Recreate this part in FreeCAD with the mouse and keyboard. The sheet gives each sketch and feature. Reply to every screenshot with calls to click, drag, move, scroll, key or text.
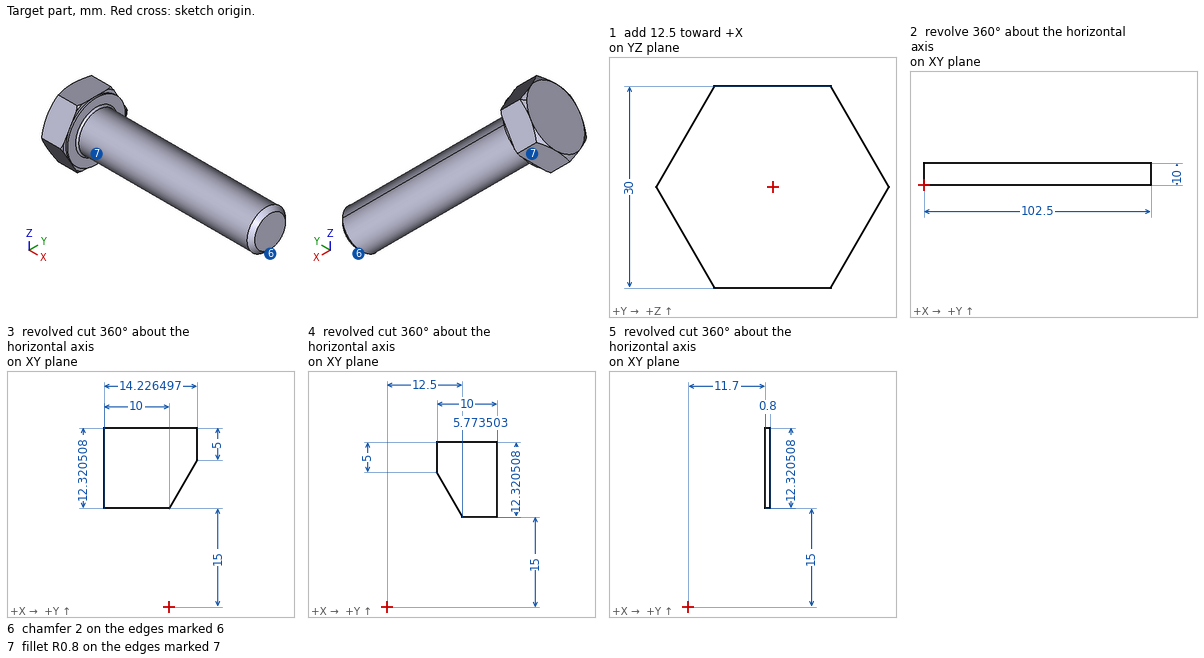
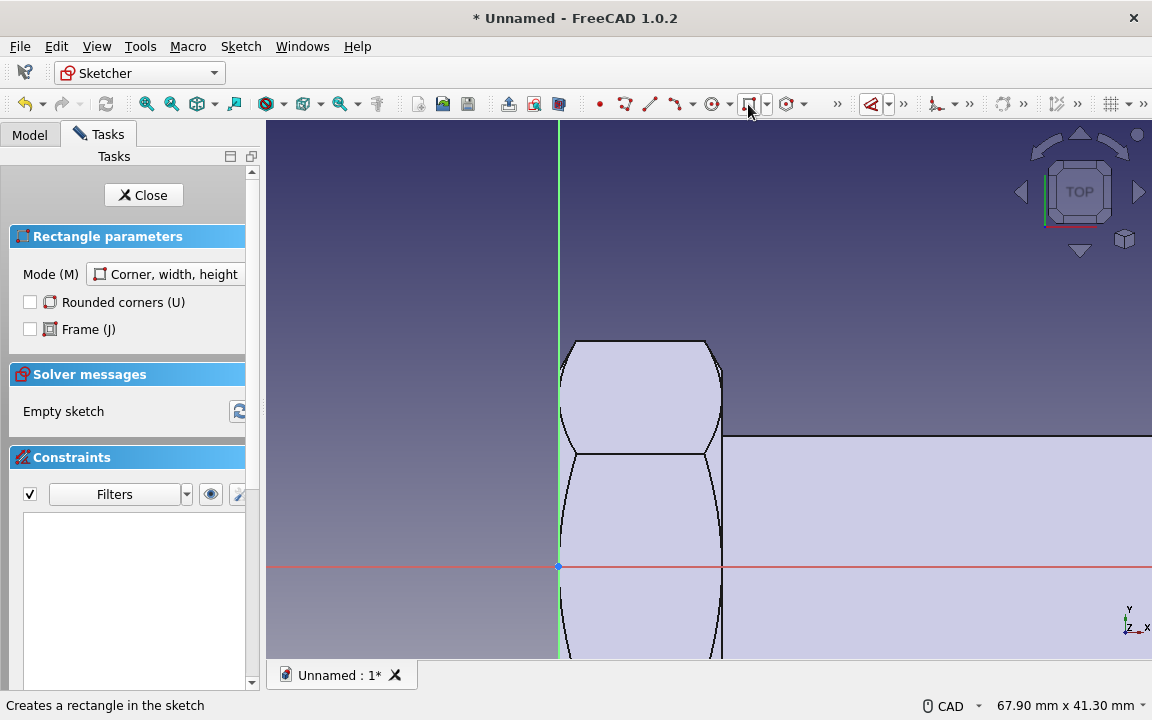
scroll(712, 210, up, 3)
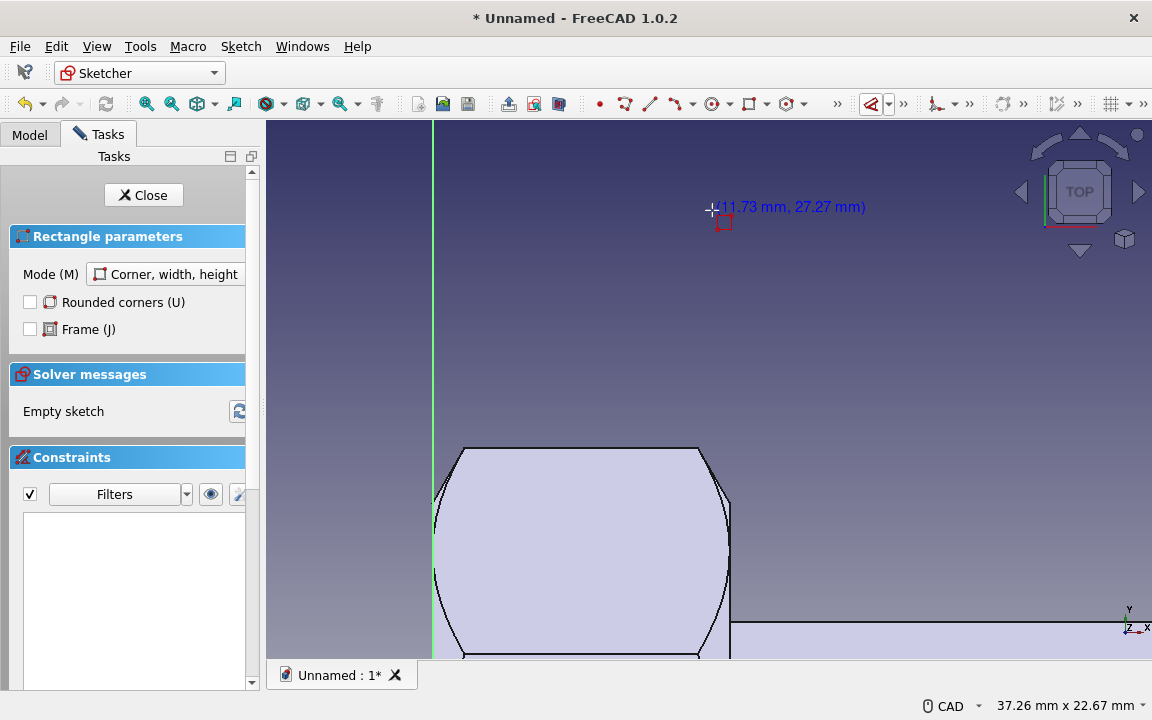
click(711, 210)
move(730, 503)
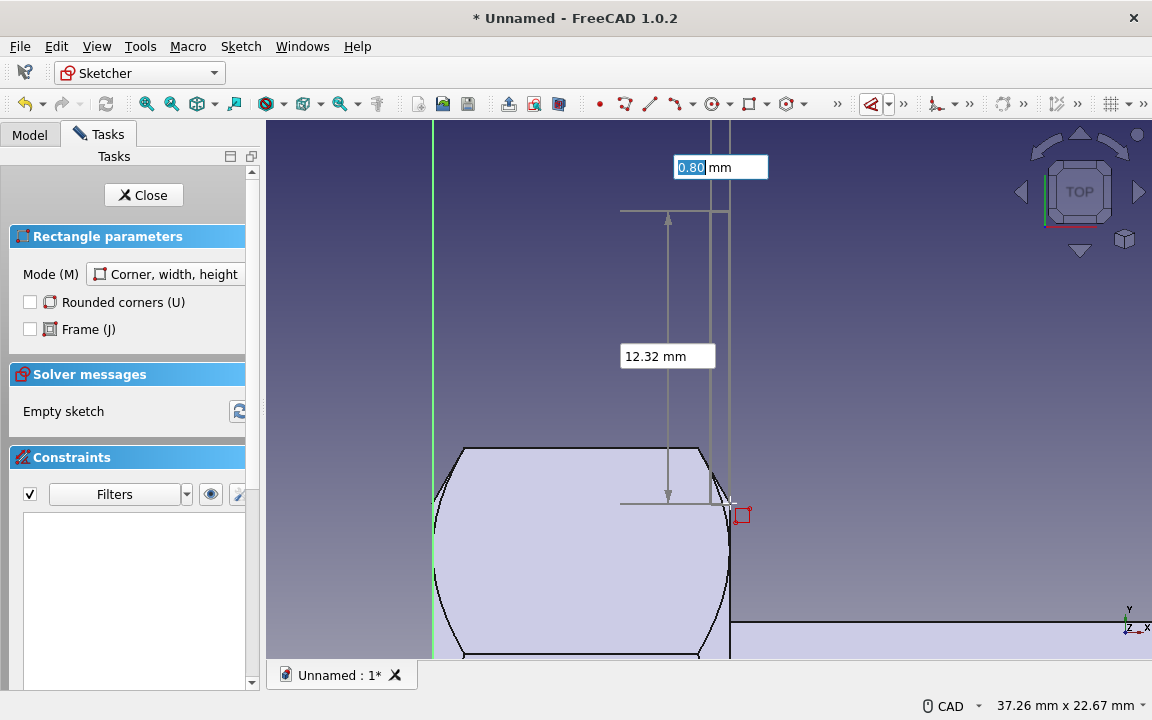
text(0.8)
key(Tab)
text(12.320508)
key(Return)
key(Escape)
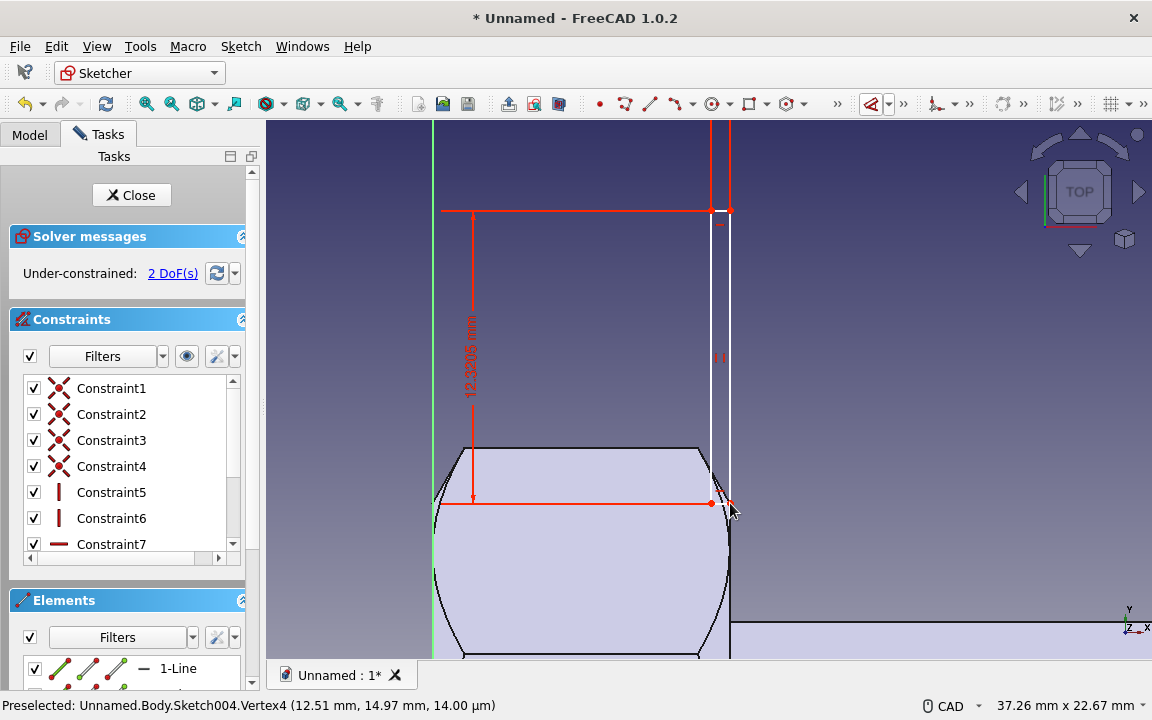
click(711, 504)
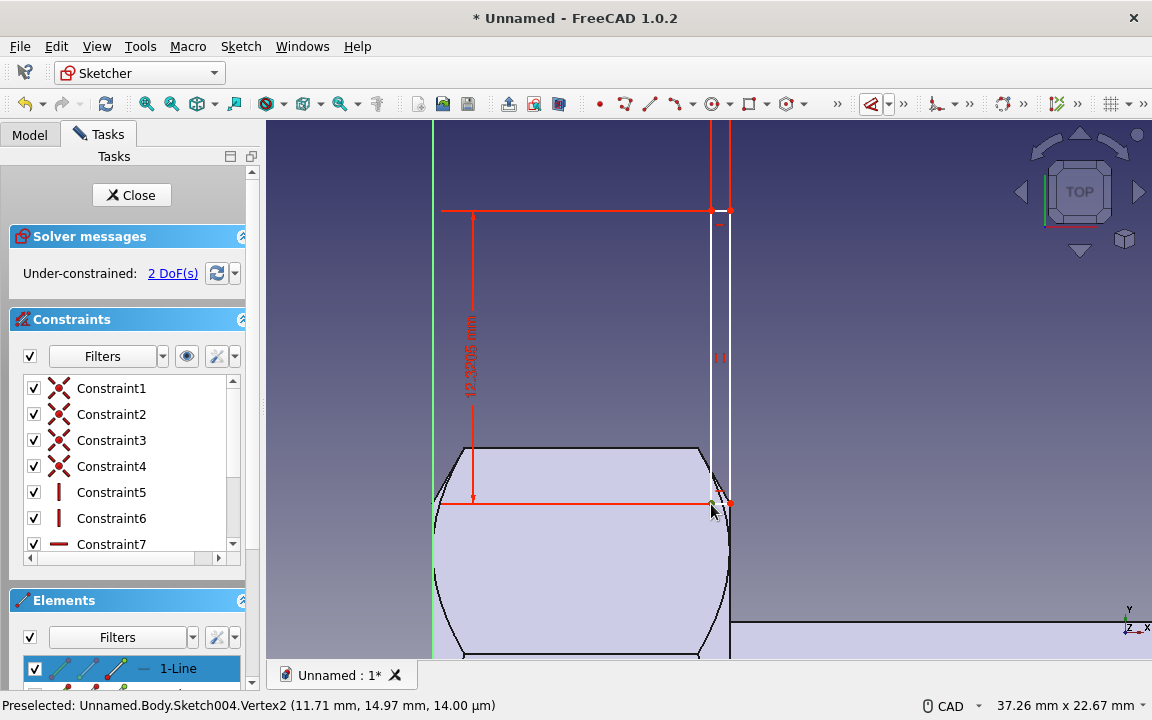
click(888, 104)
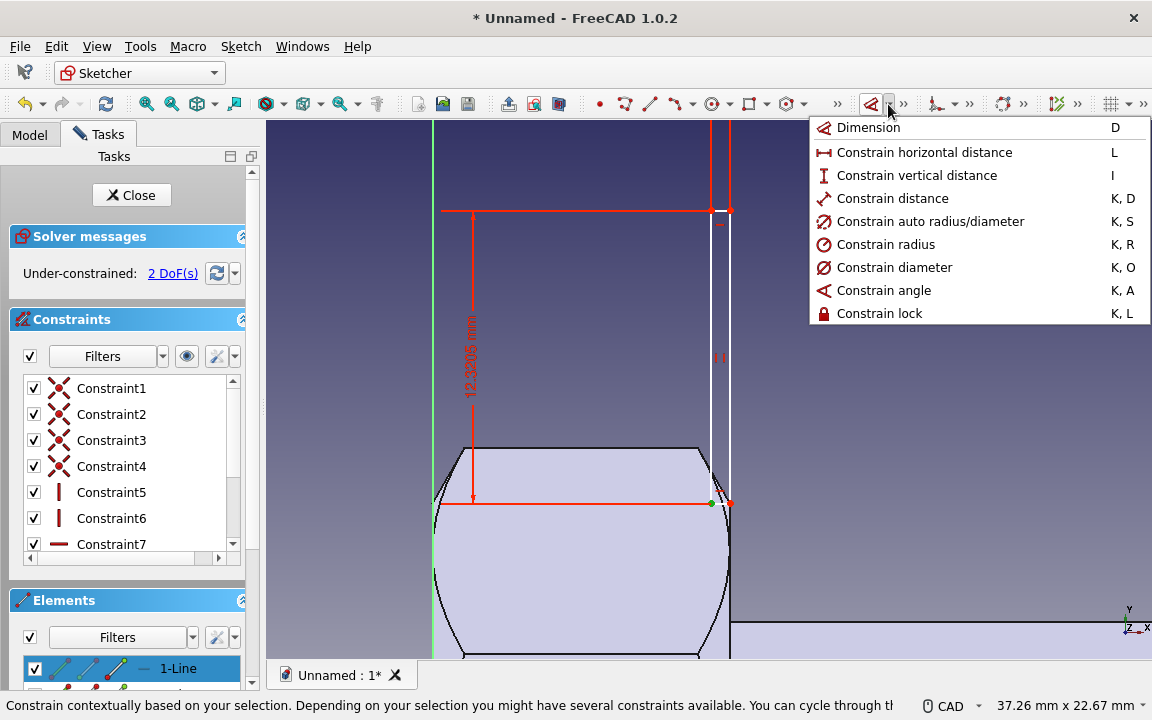
click(980, 176)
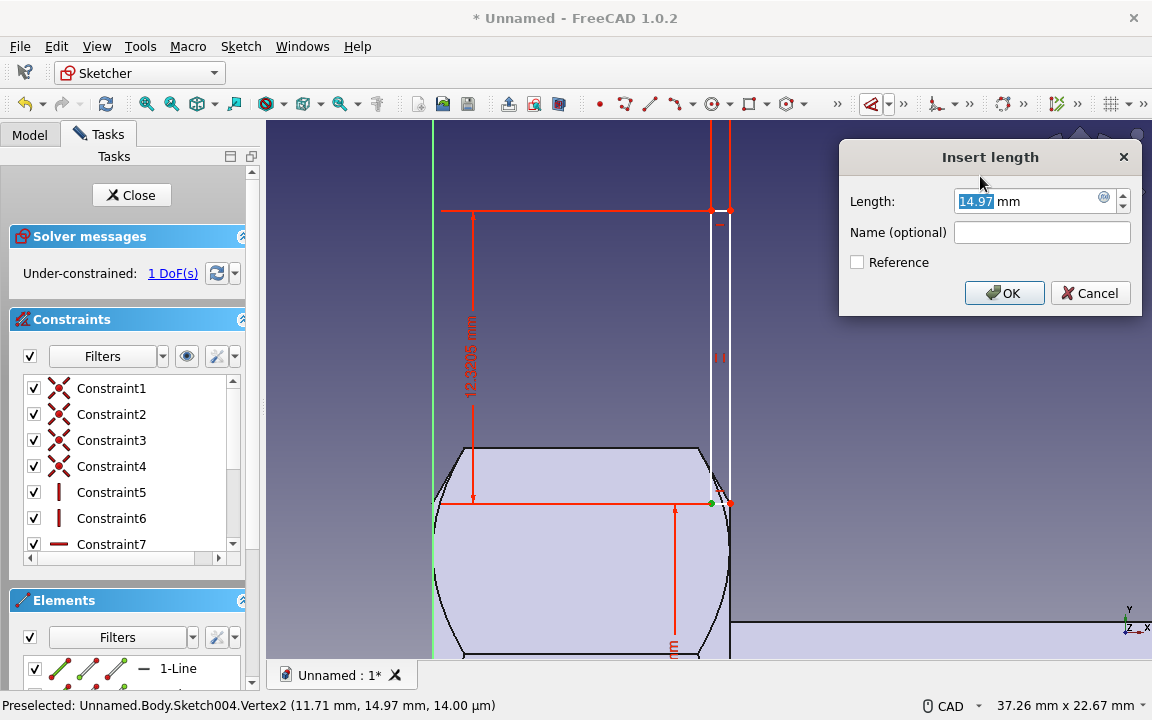
text(15)
key(Return)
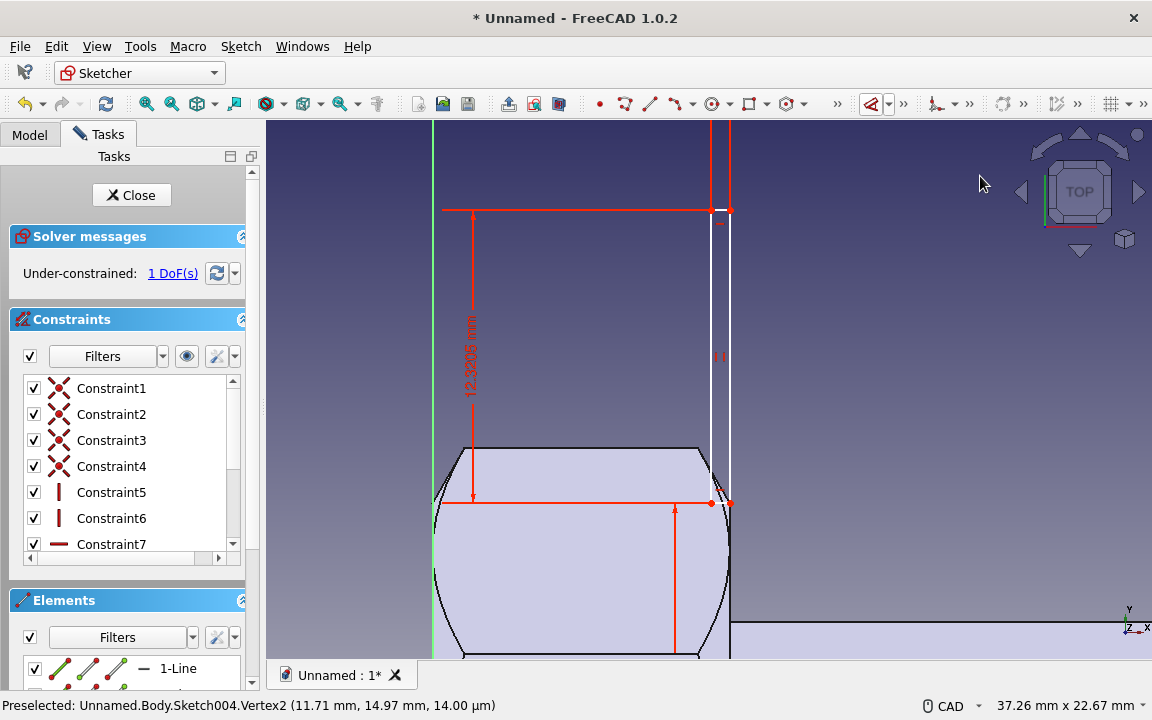
click(711, 210)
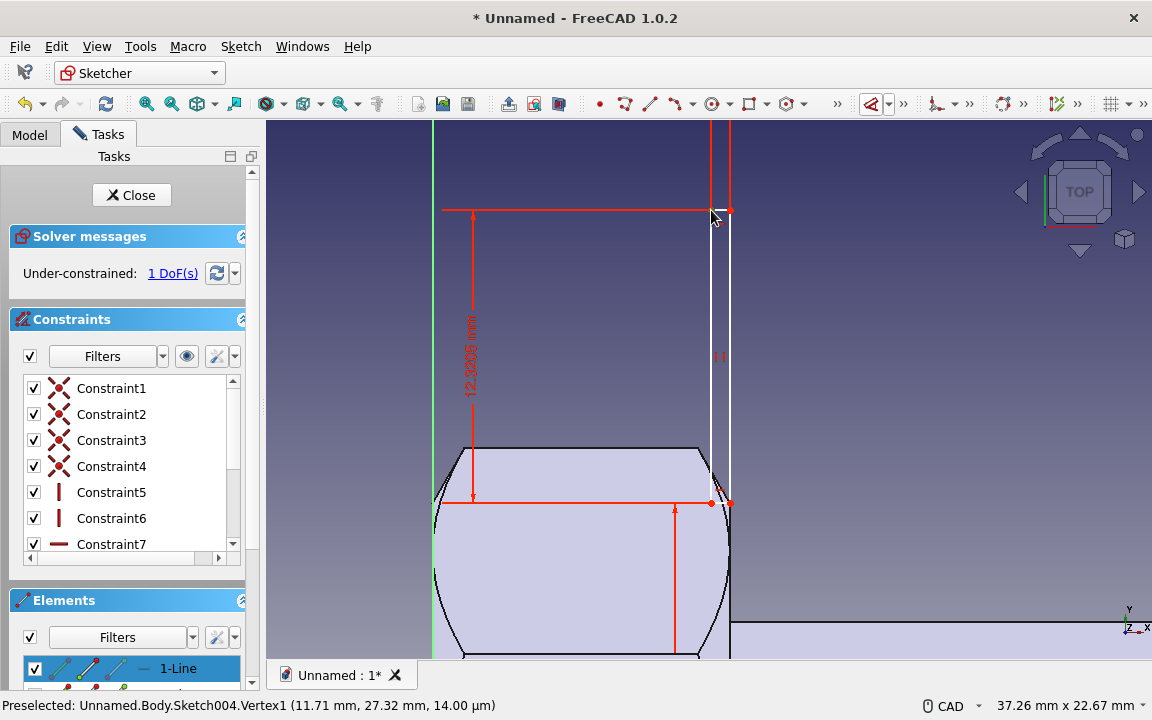
click(888, 104)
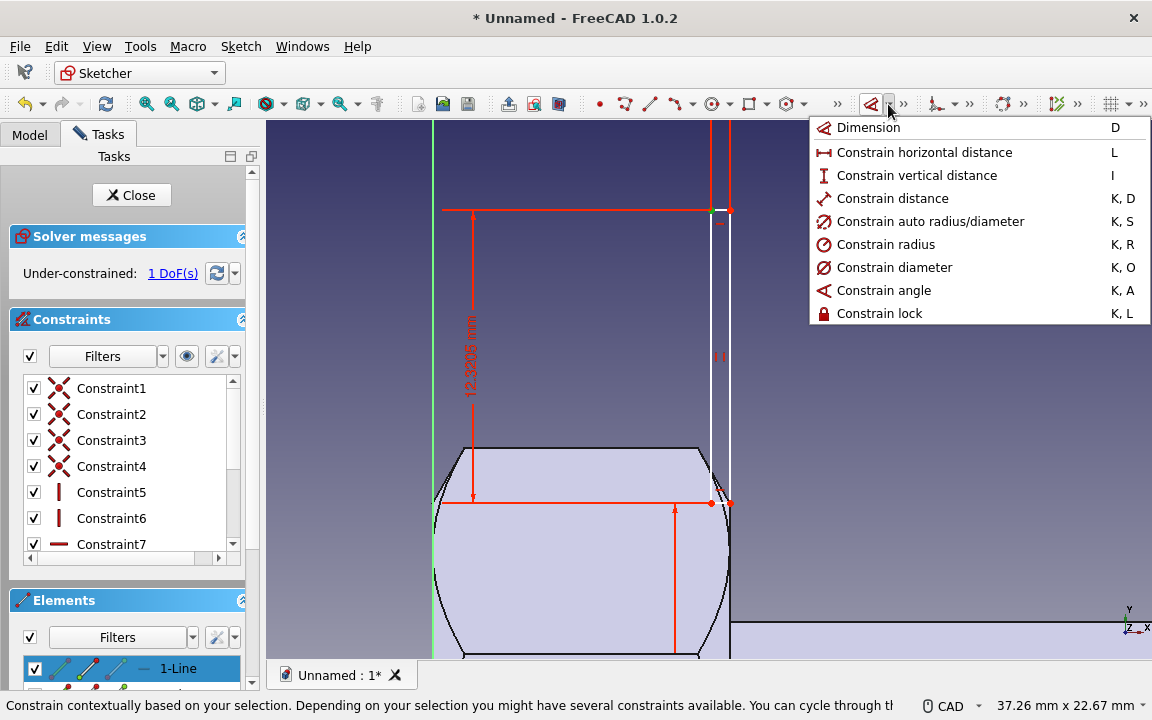
click(980, 152)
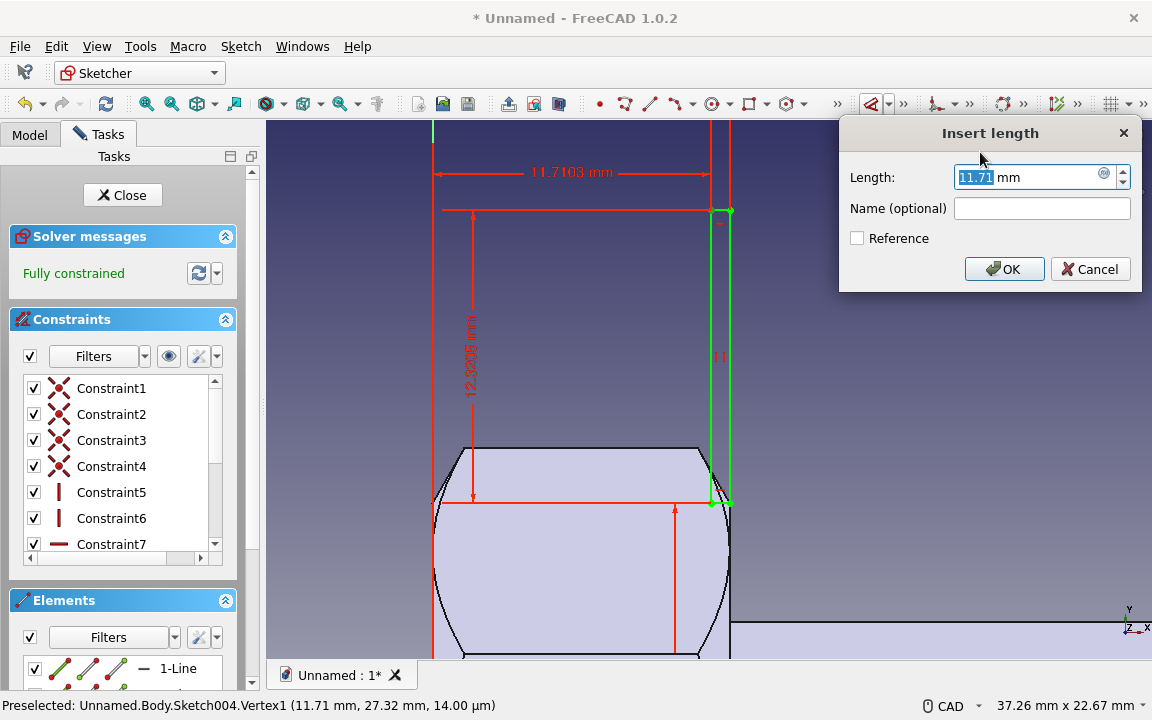
text(11.7)
key(Return)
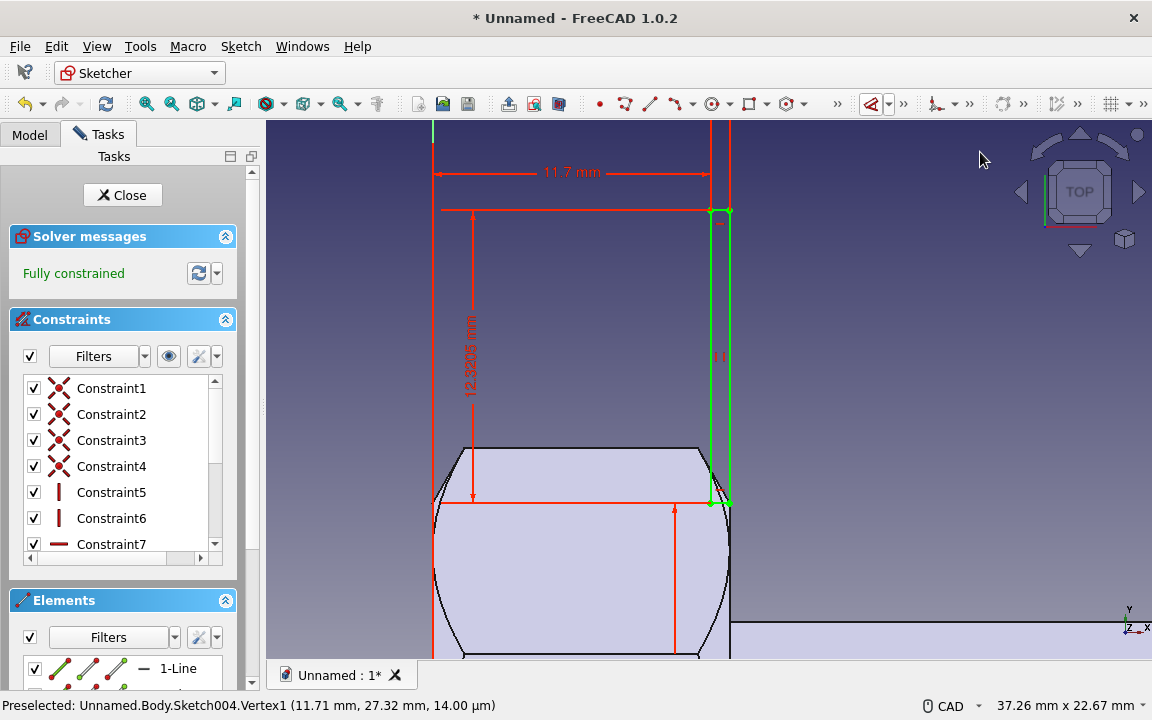
click(123, 195)